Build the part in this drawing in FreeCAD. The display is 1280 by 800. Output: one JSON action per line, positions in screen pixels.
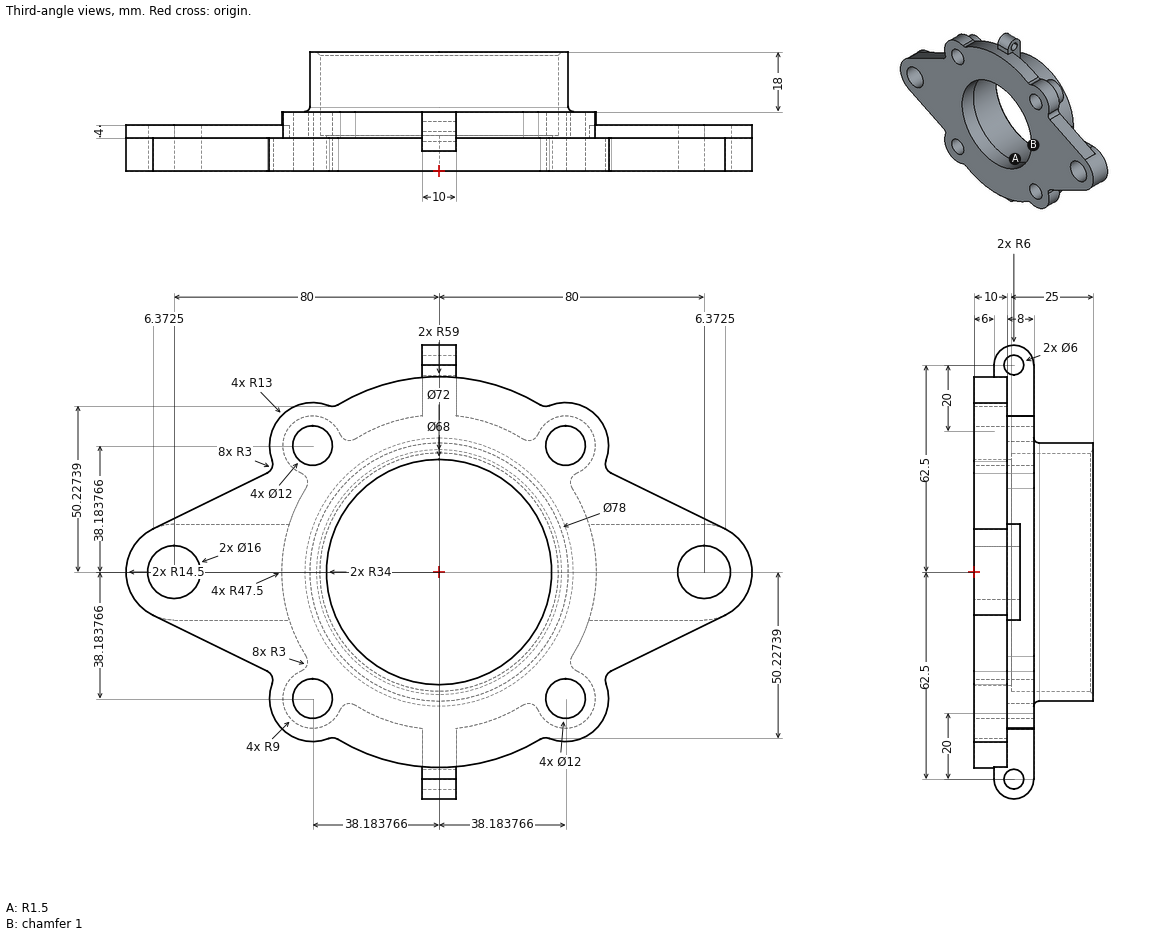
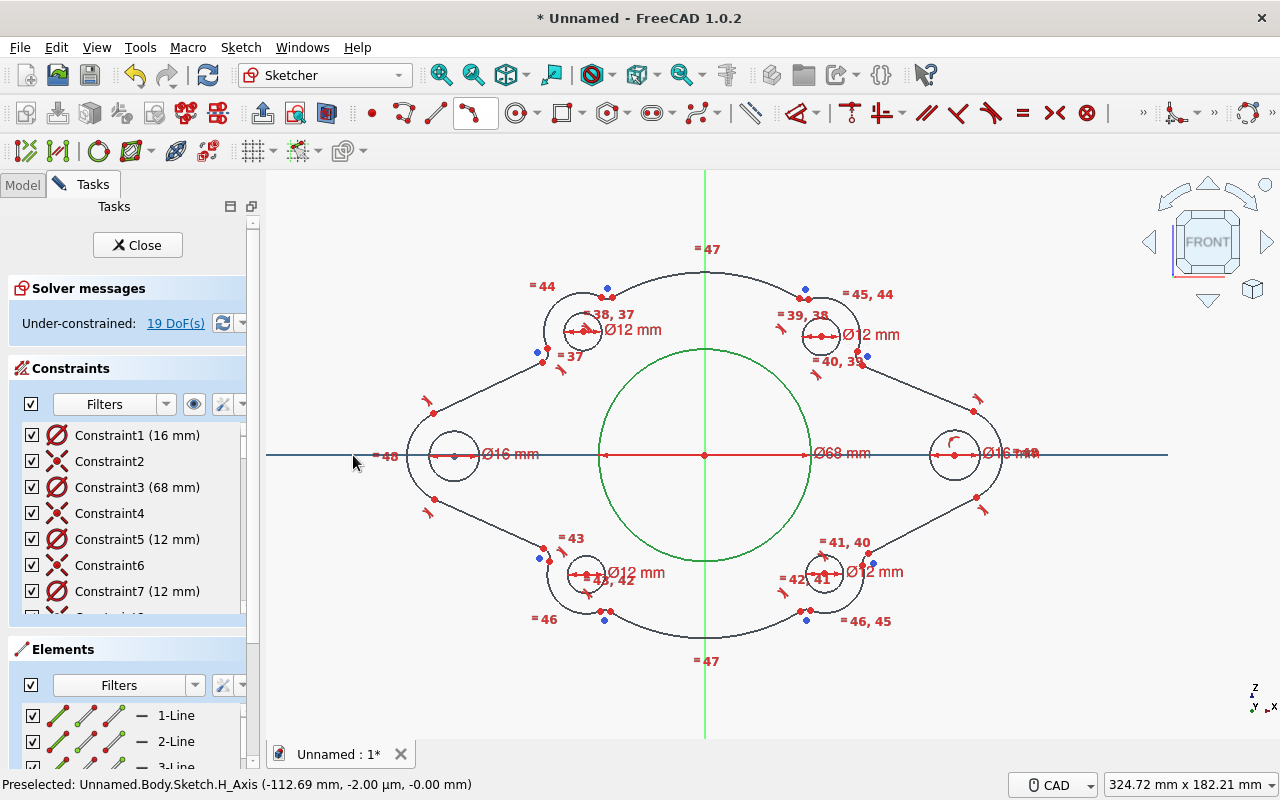
{"action": "left_click", "coordinate": [850, 114]}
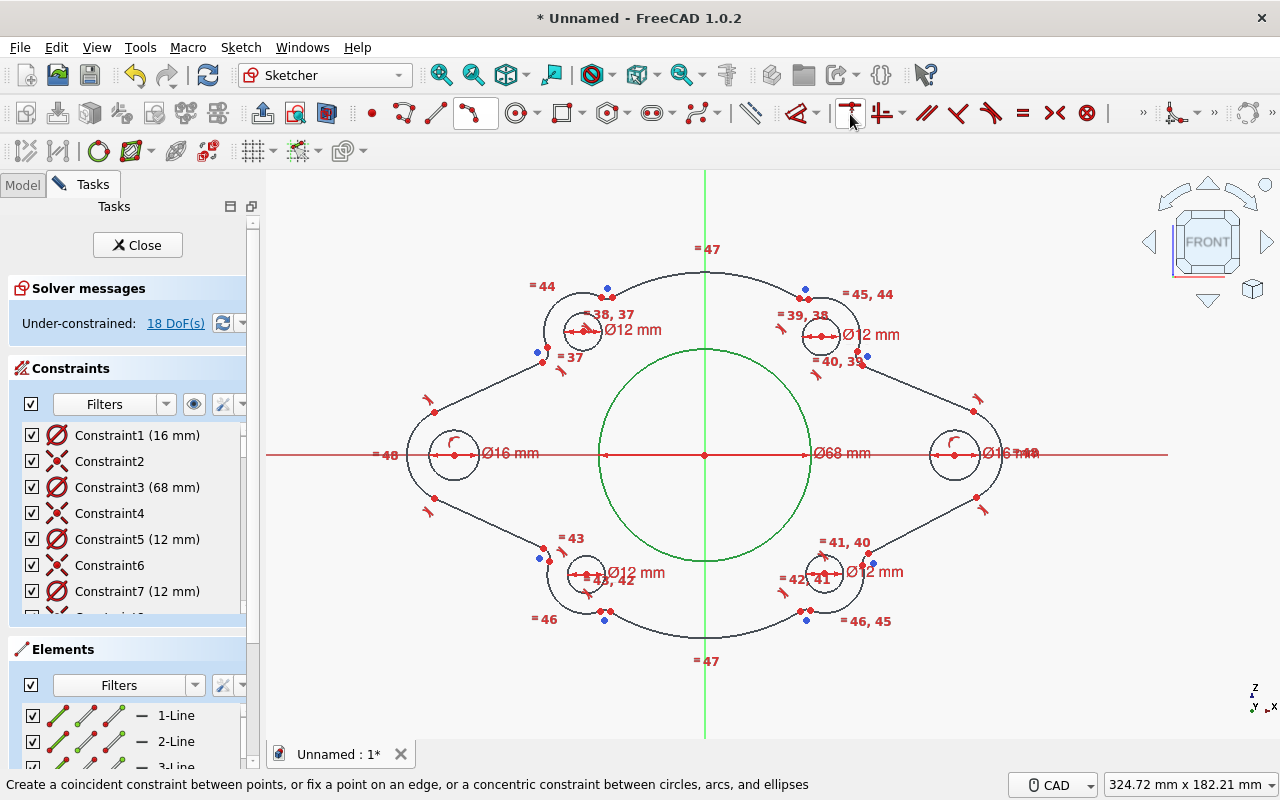
{"action": "left_click", "coordinate": [796, 114]}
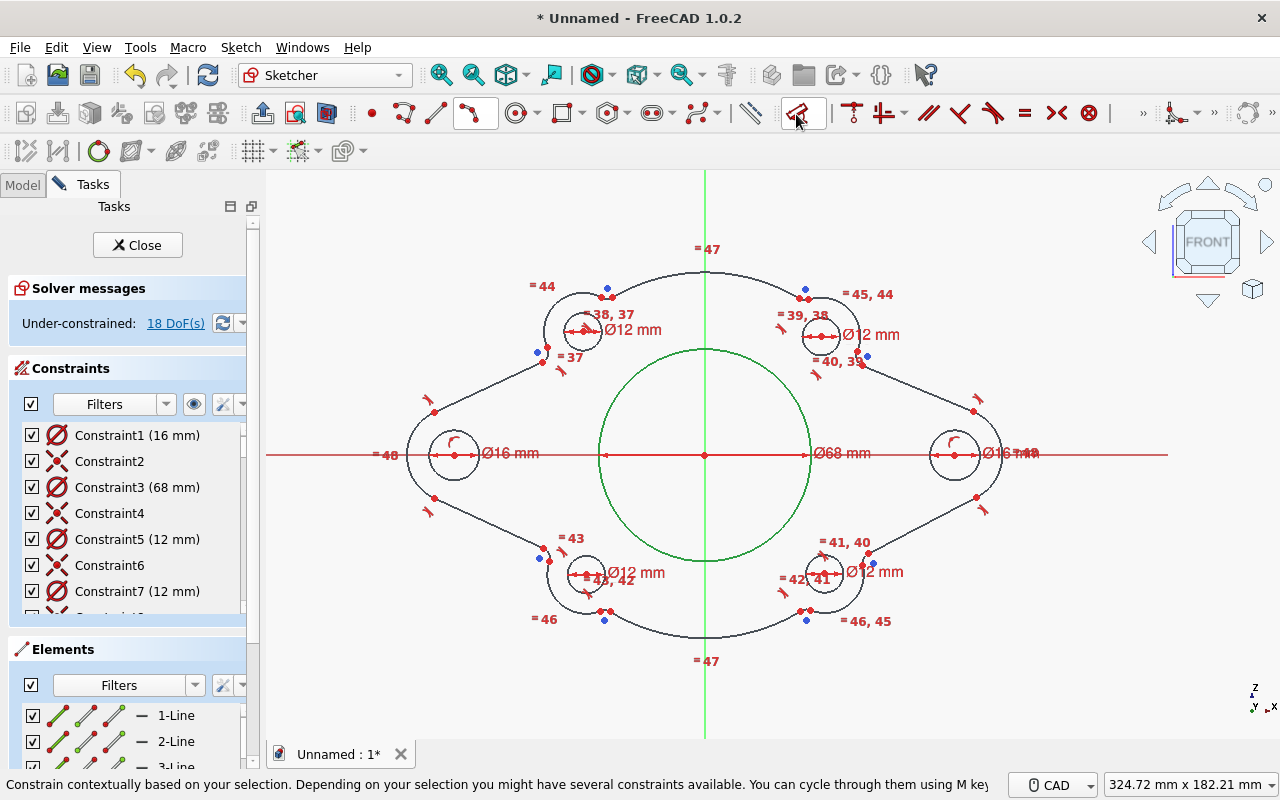
{"action": "scroll", "coordinate": [548, 356], "scroll_direction": "up", "scroll_amount": 8}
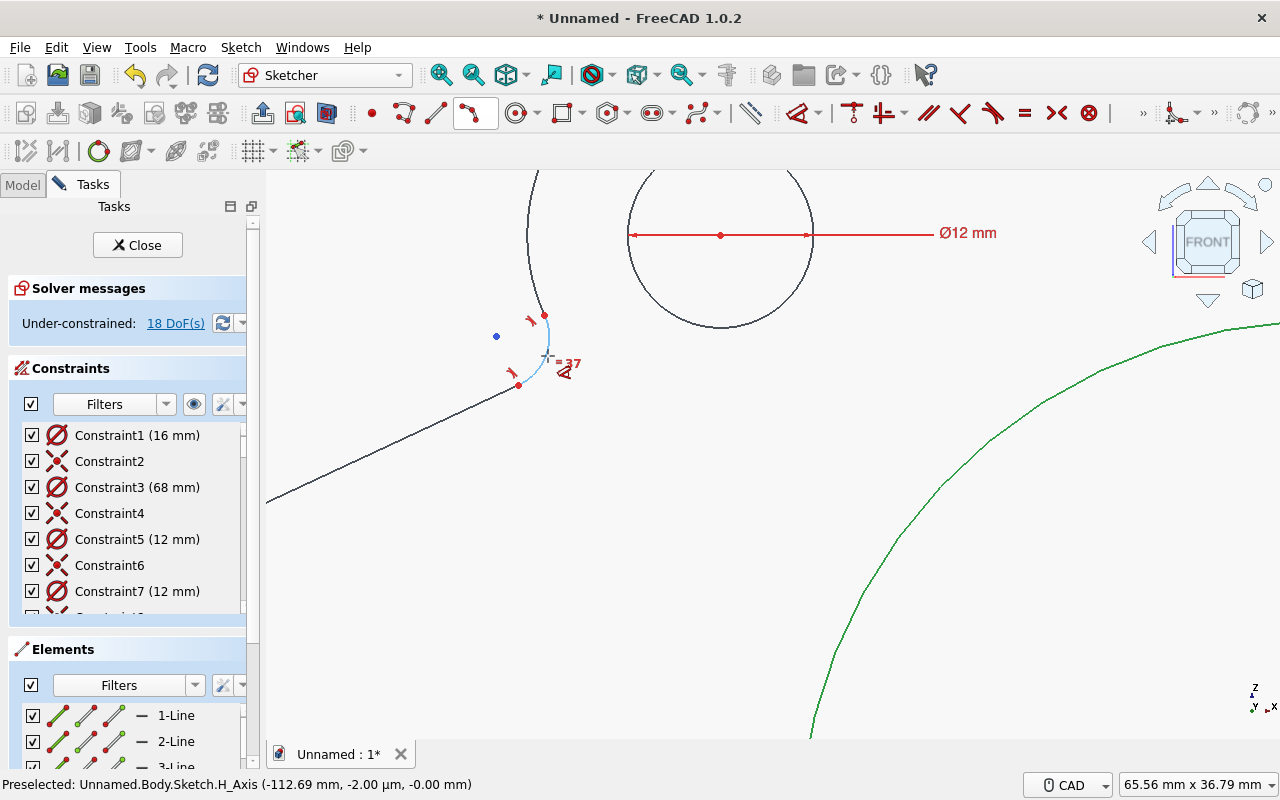
{"action": "left_click", "coordinate": [546, 355]}
{"action": "left_click", "coordinate": [576, 366]}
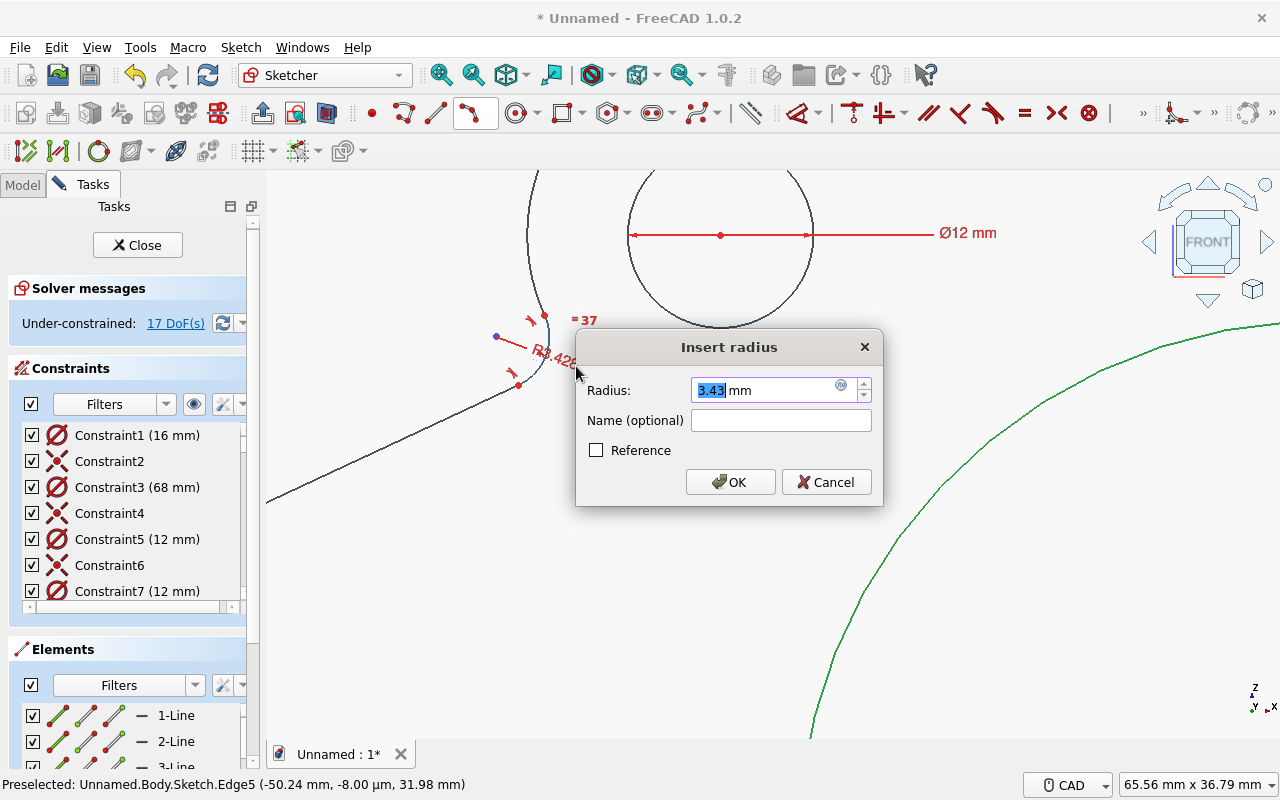
{"action": "type", "text": "3"}
{"action": "key", "text": "Return"}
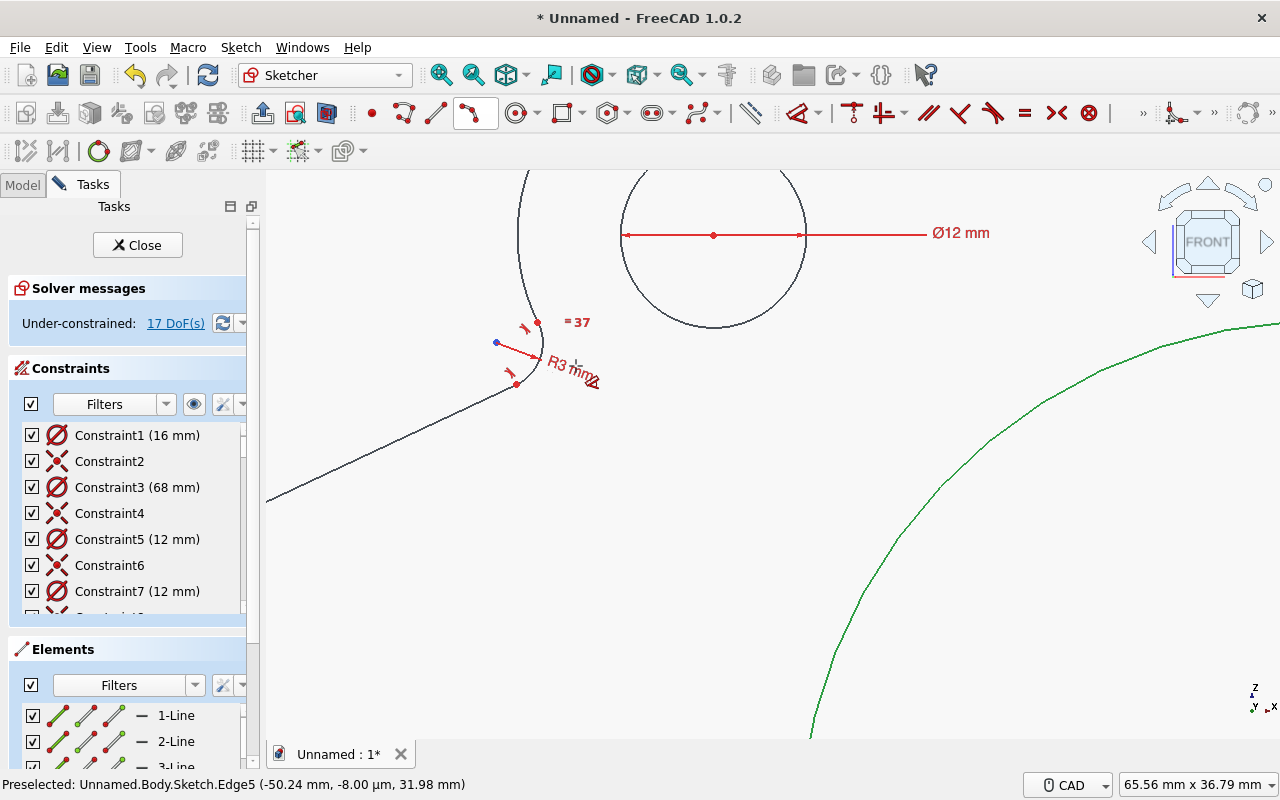
{"action": "scroll", "coordinate": [548, 355], "scroll_direction": "down", "scroll_amount": 8}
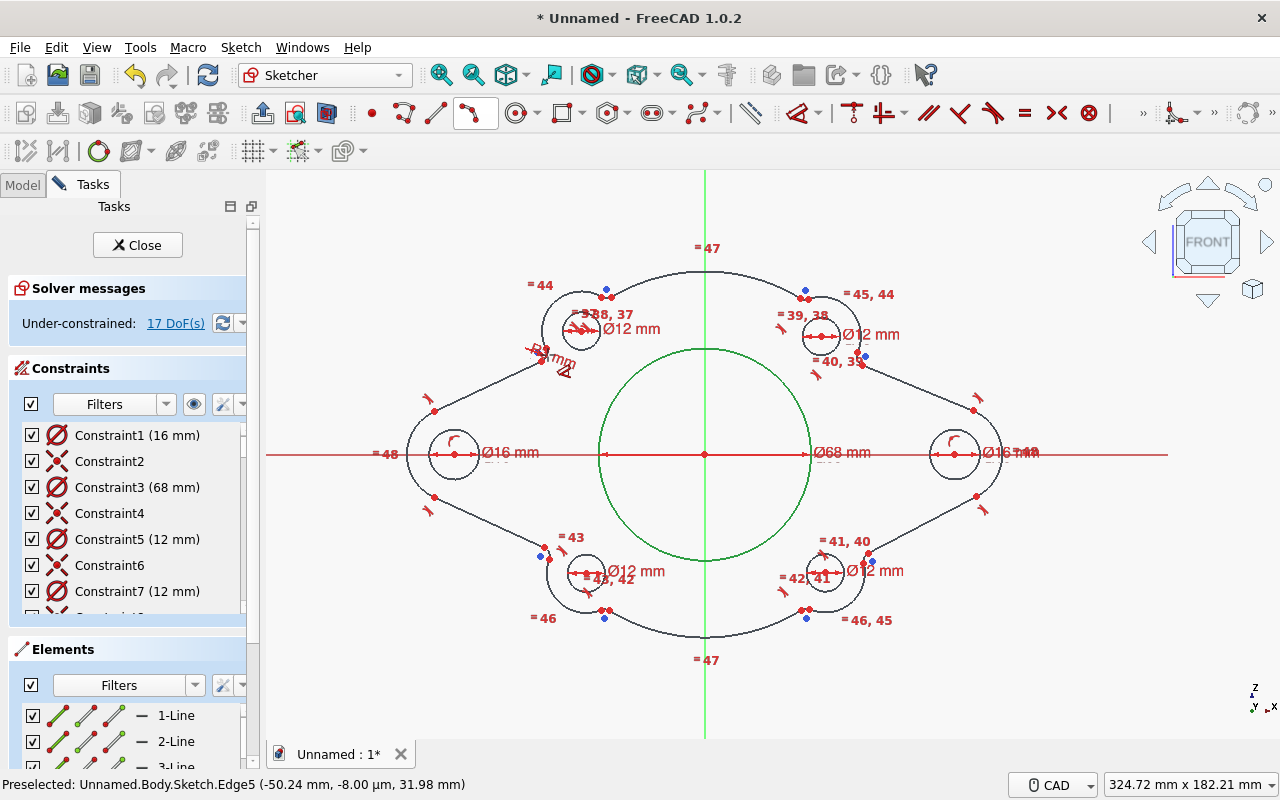
{"action": "left_click", "coordinate": [542, 329]}
{"action": "left_click", "coordinate": [510, 327]}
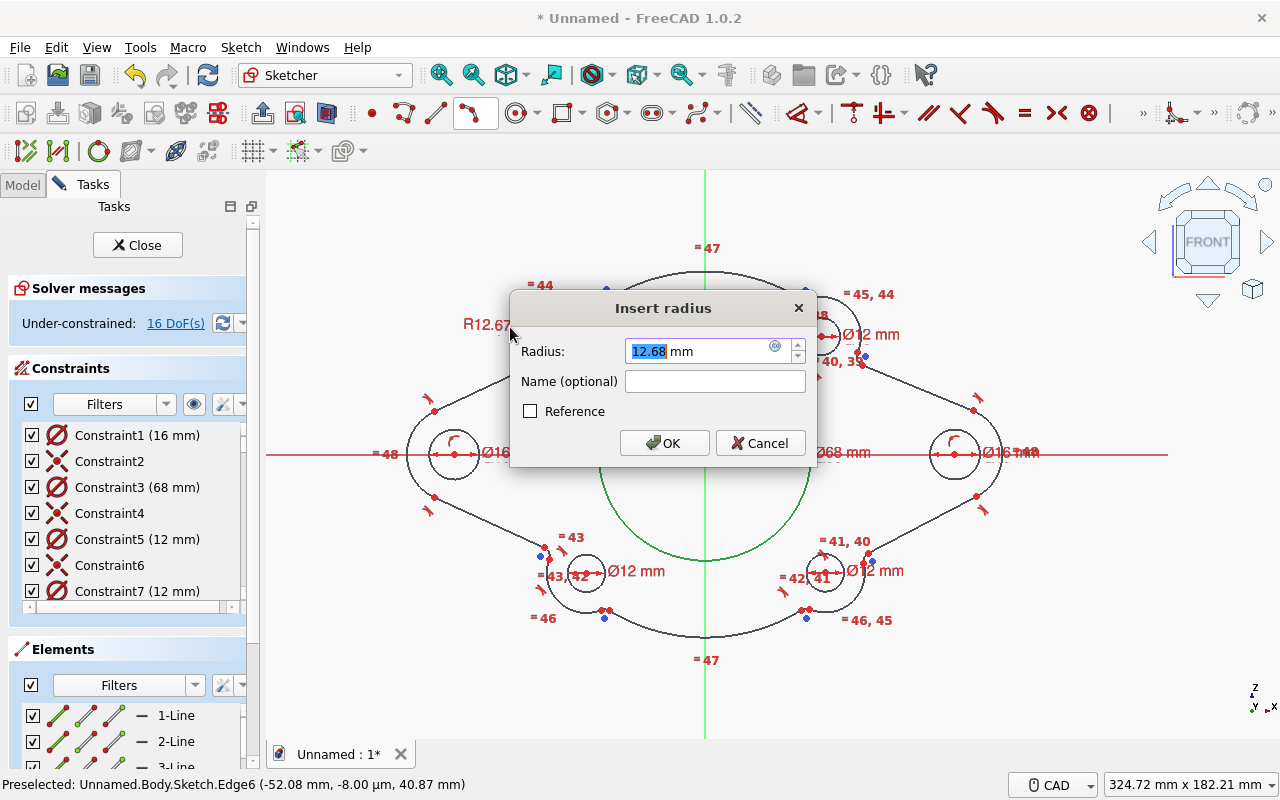
{"action": "type", "text": "13"}
{"action": "key", "text": "Return"}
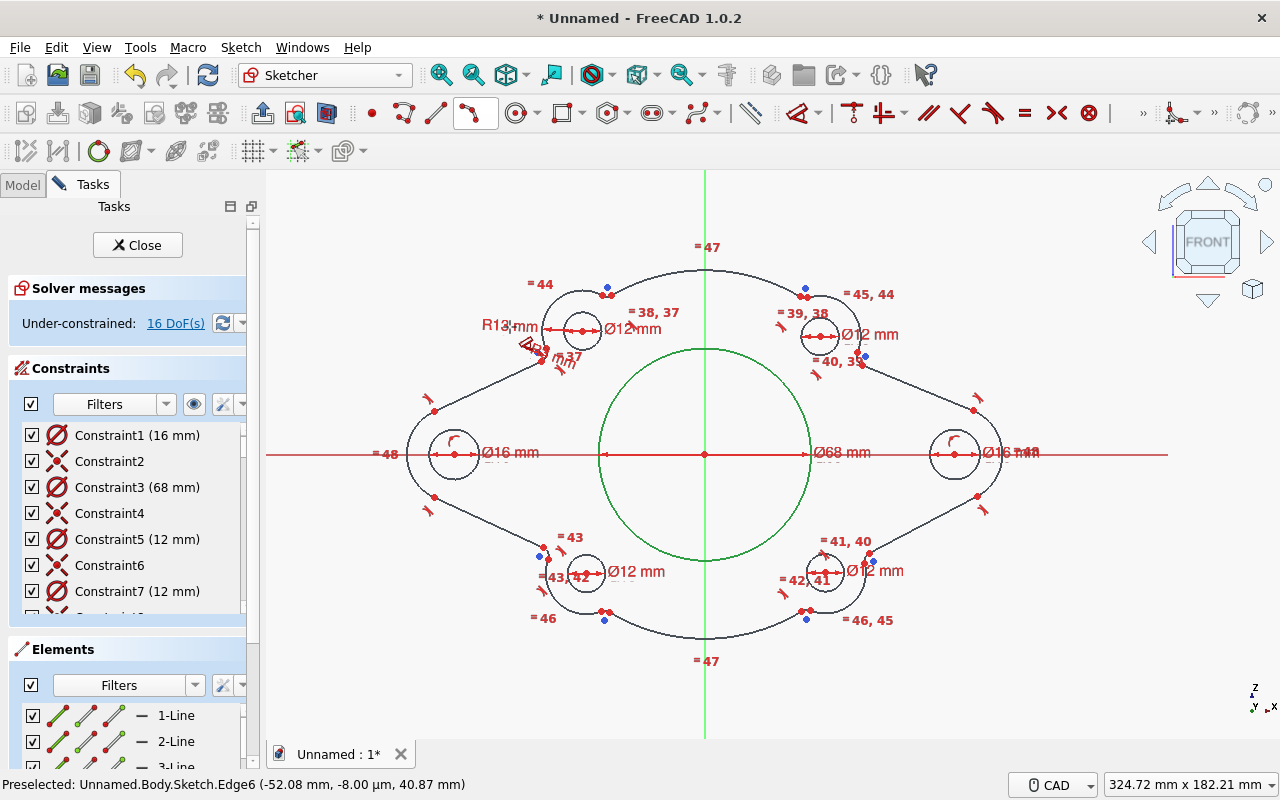
{"action": "left_click", "coordinate": [745, 275]}
{"action": "left_click", "coordinate": [752, 244]}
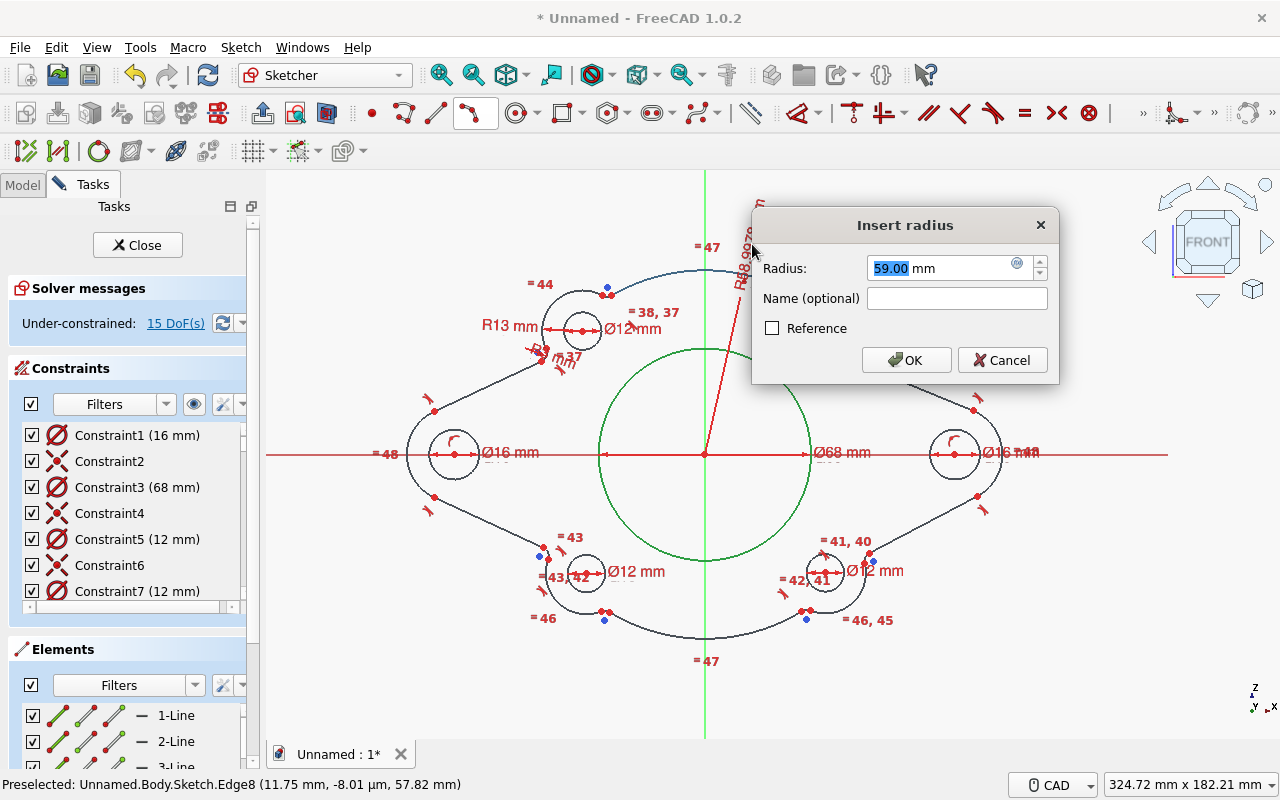
{"action": "type", "text": "59"}
{"action": "key", "text": "Return"}